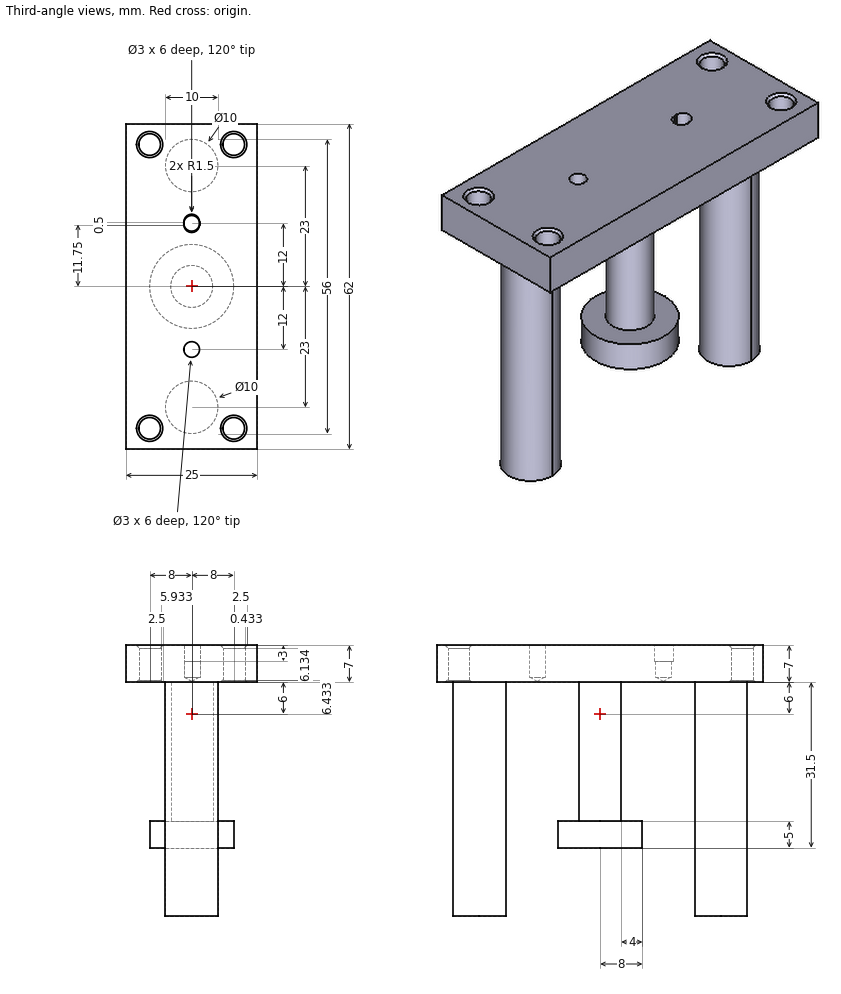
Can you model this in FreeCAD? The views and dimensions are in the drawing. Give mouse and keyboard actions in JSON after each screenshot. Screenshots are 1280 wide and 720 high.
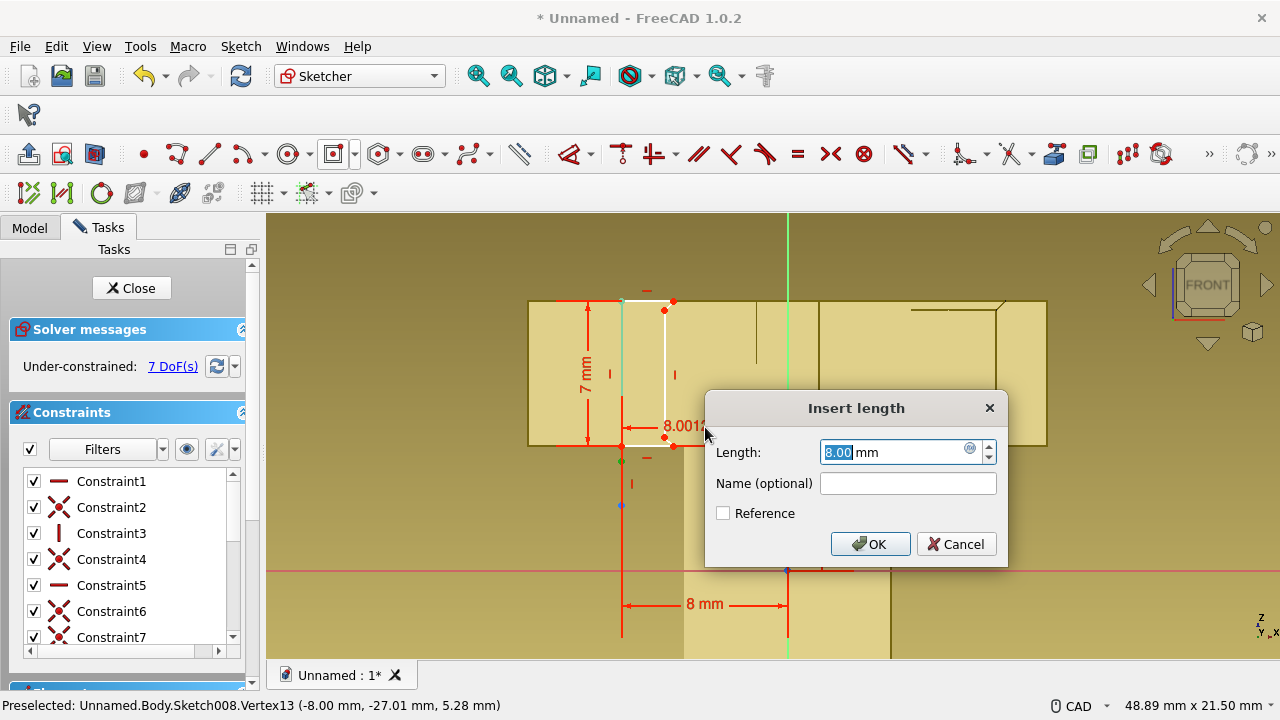
{"action": "type", "text": "8"}
{"action": "key", "text": "Return"}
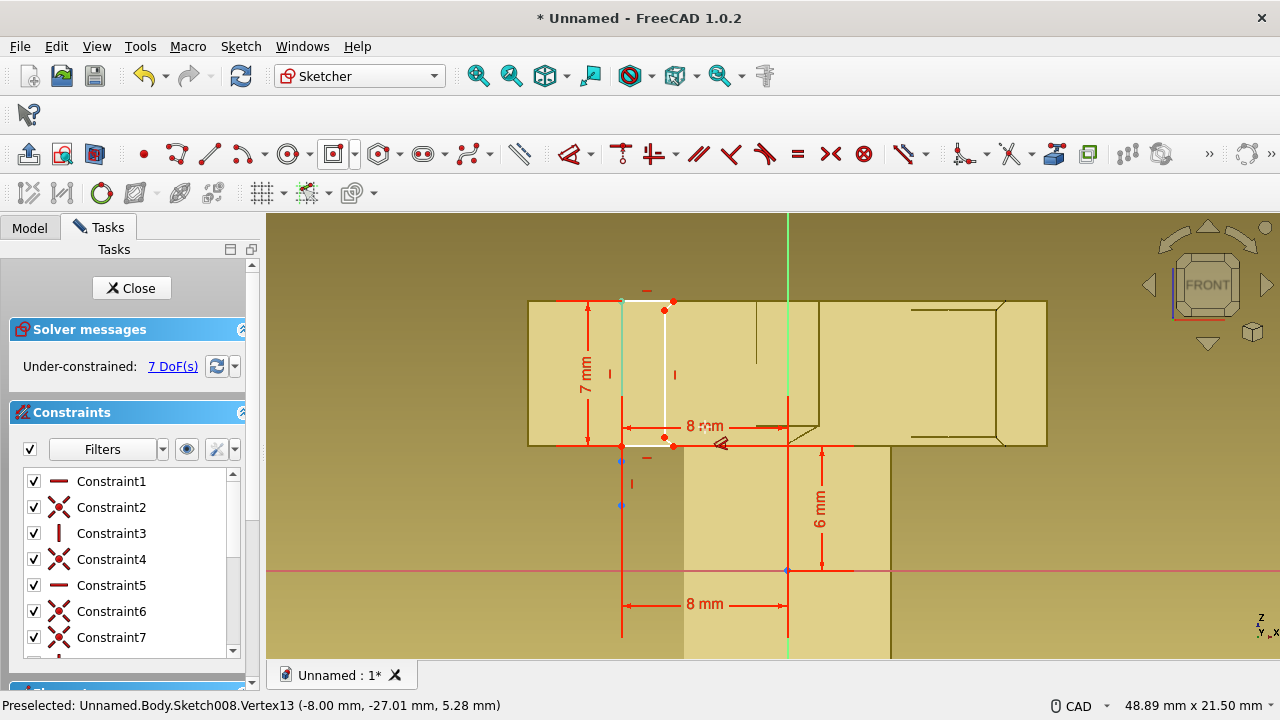
{"action": "scroll", "coordinate": [658, 446], "scroll_direction": "up", "scroll_amount": 2}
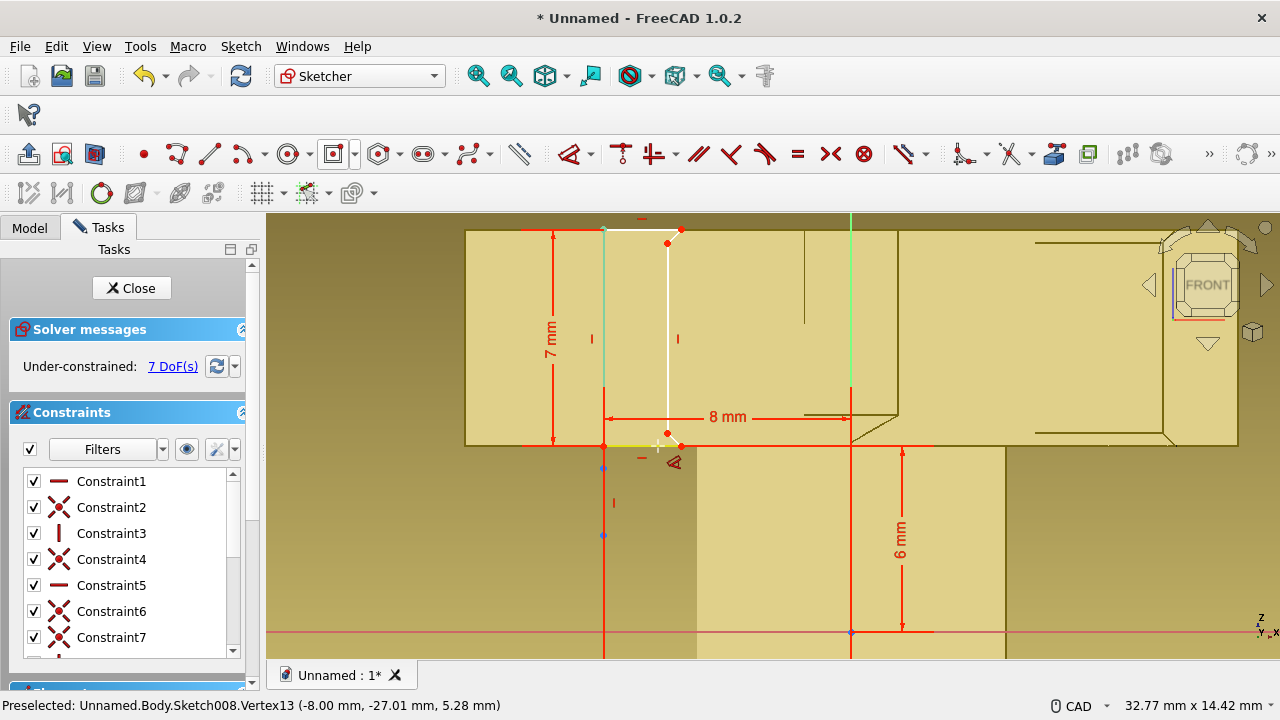
{"action": "left_click", "coordinate": [658, 446]}
{"action": "left_click", "coordinate": [643, 480]}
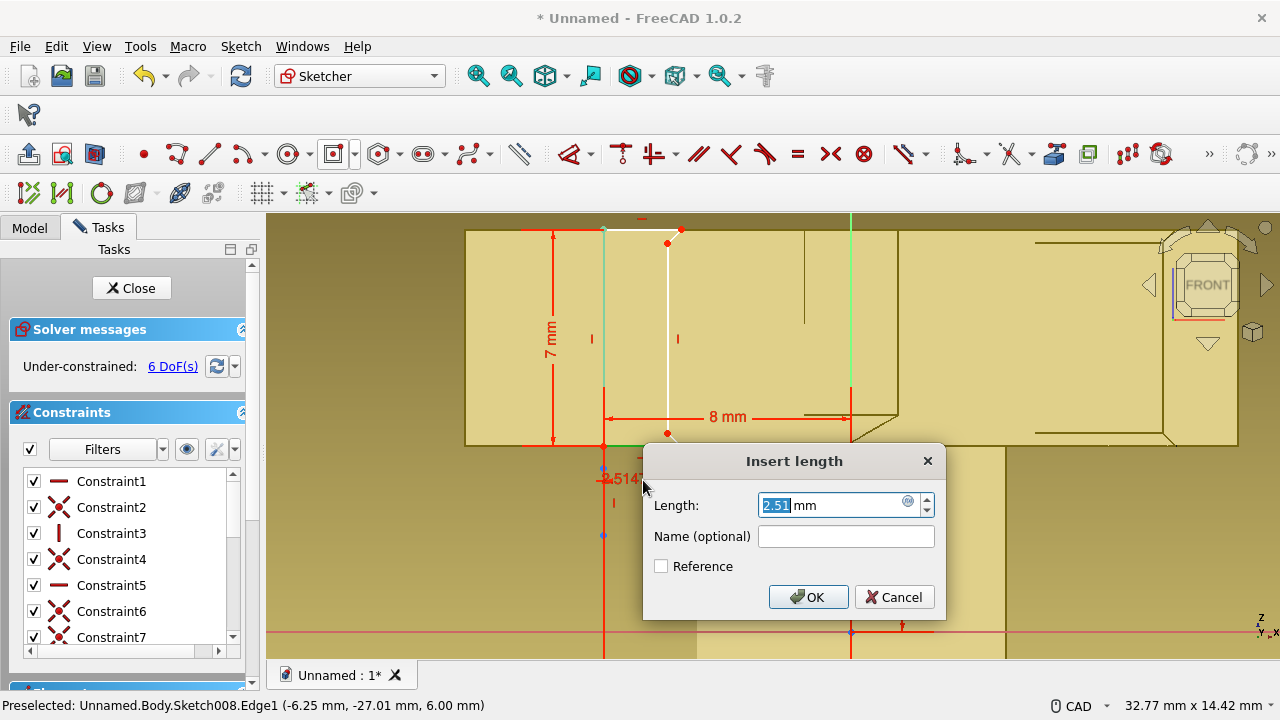
{"action": "type", "text": "2.5"}
{"action": "key", "text": "Return"}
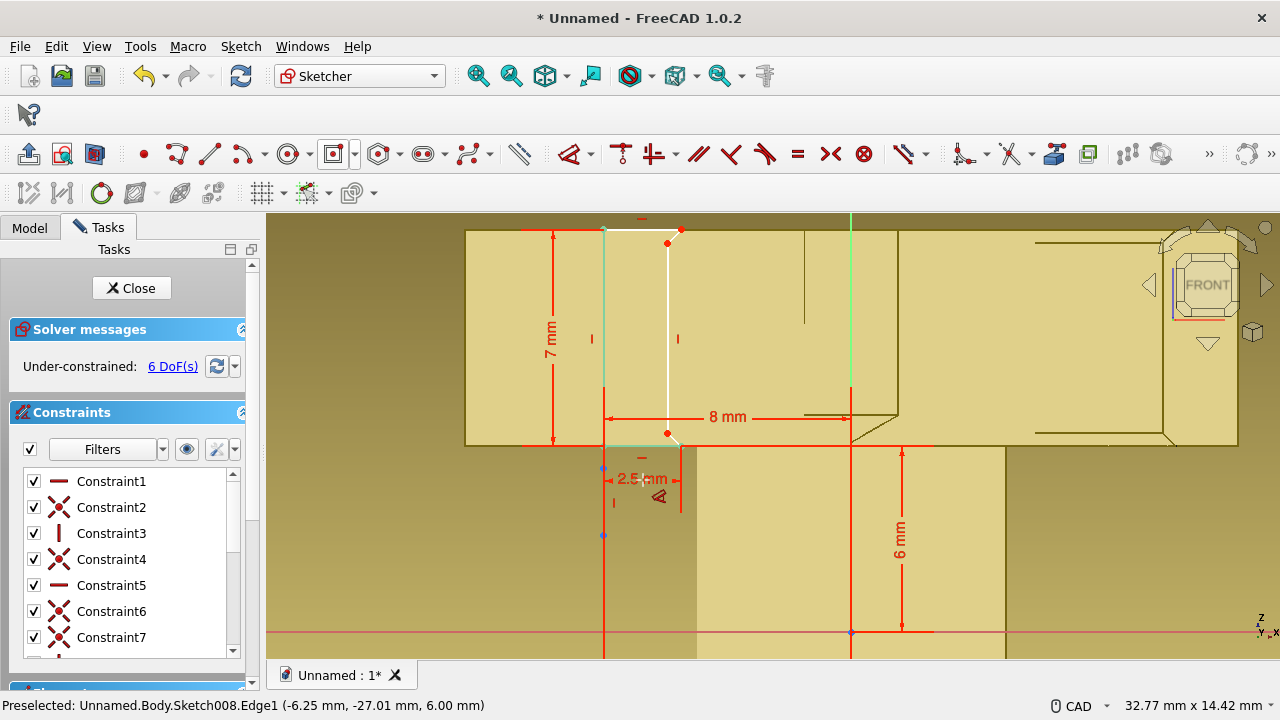
{"action": "scroll", "coordinate": [658, 446], "scroll_direction": "down", "scroll_amount": 2}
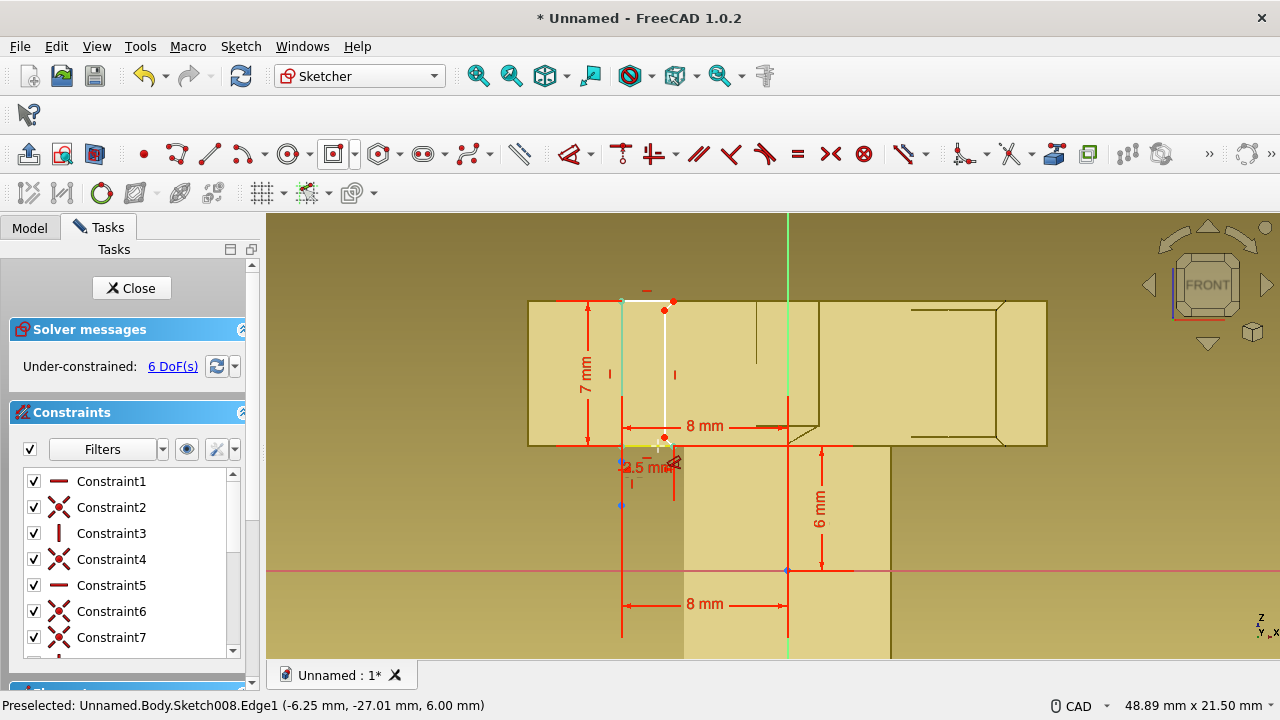
{"action": "left_click", "coordinate": [637, 301]}
{"action": "left_click", "coordinate": [648, 267]}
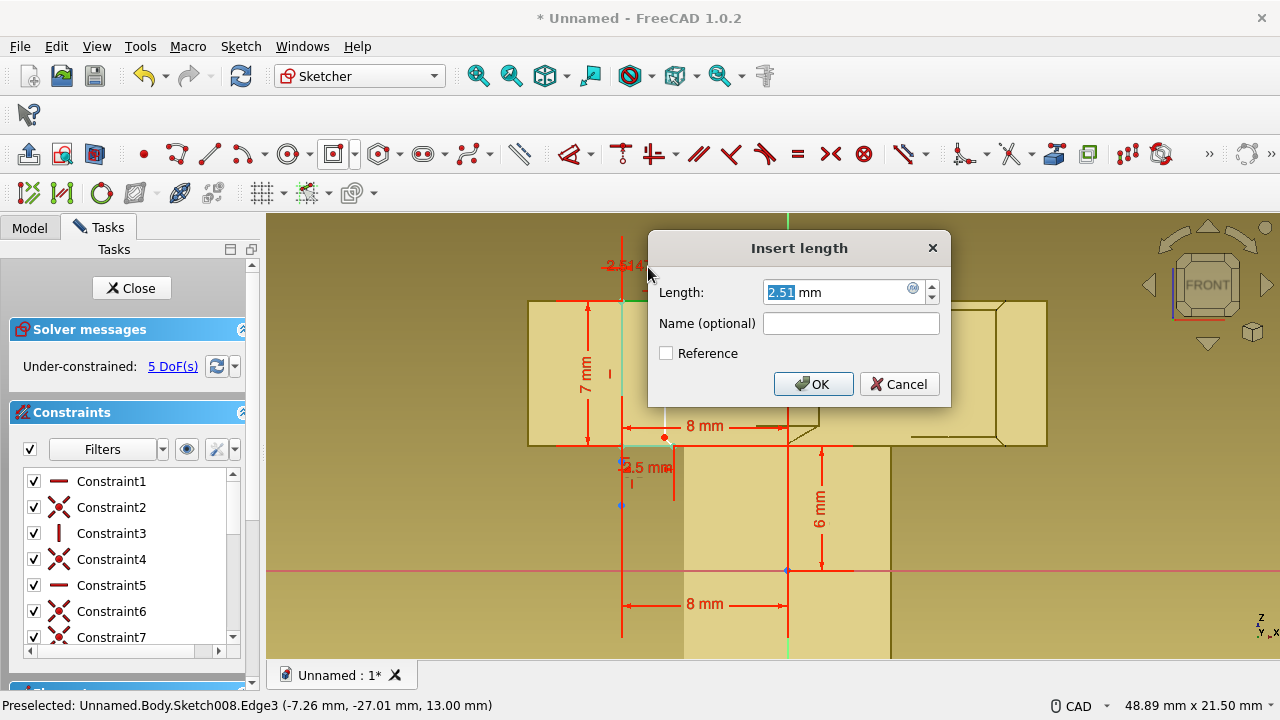
{"action": "type", "text": "2.5"}
{"action": "key", "text": "Return"}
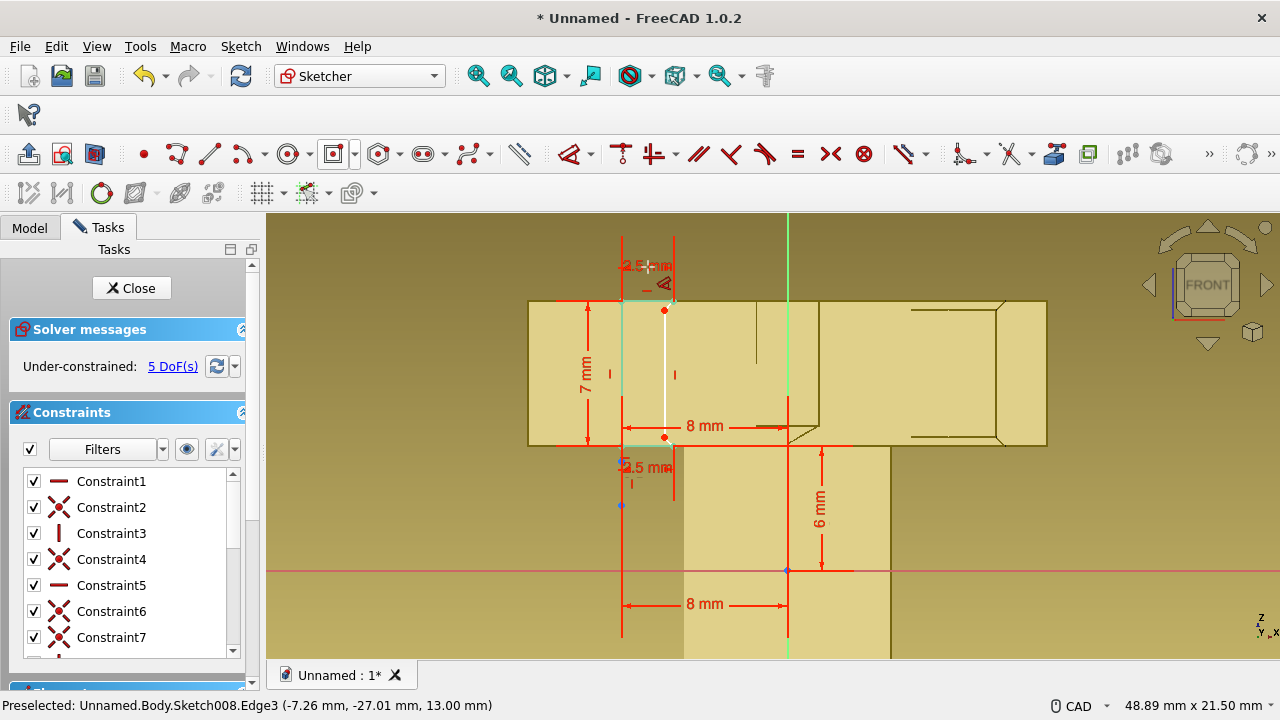
{"action": "left_click", "coordinate": [665, 349]}
{"action": "left_click", "coordinate": [699, 374]}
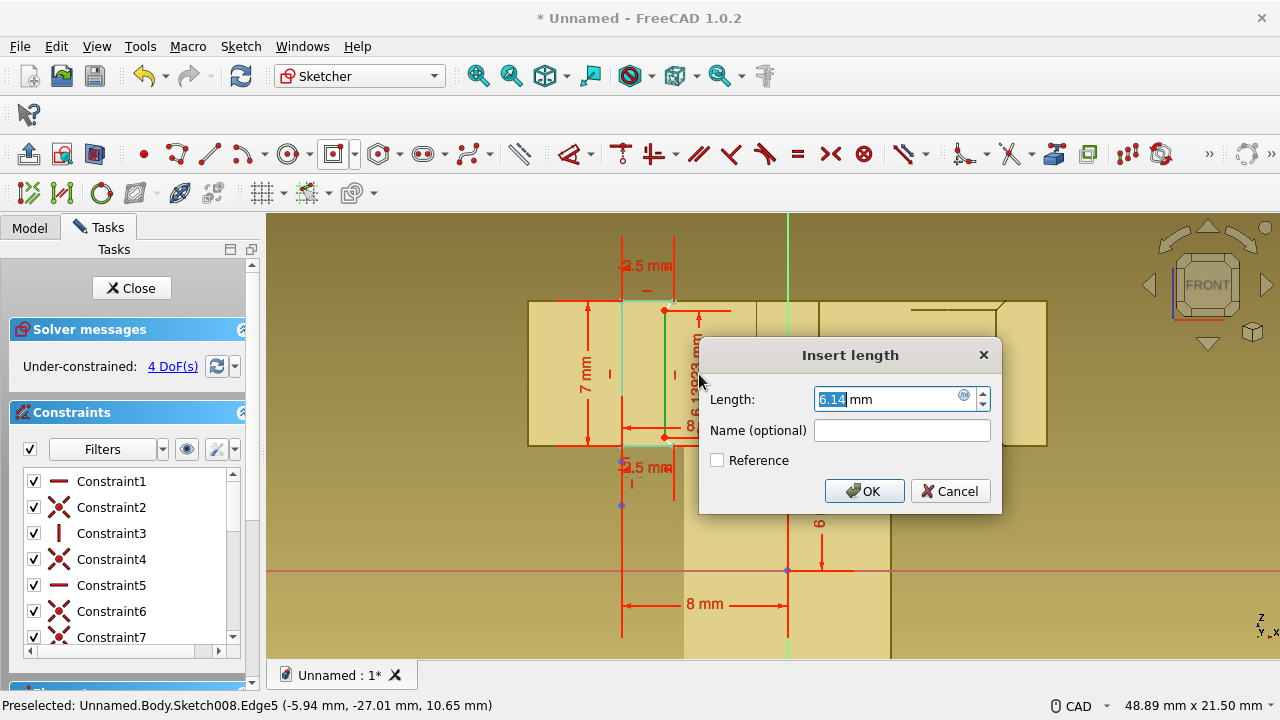
{"action": "type", "text": "6.134"}
{"action": "key", "text": "Return"}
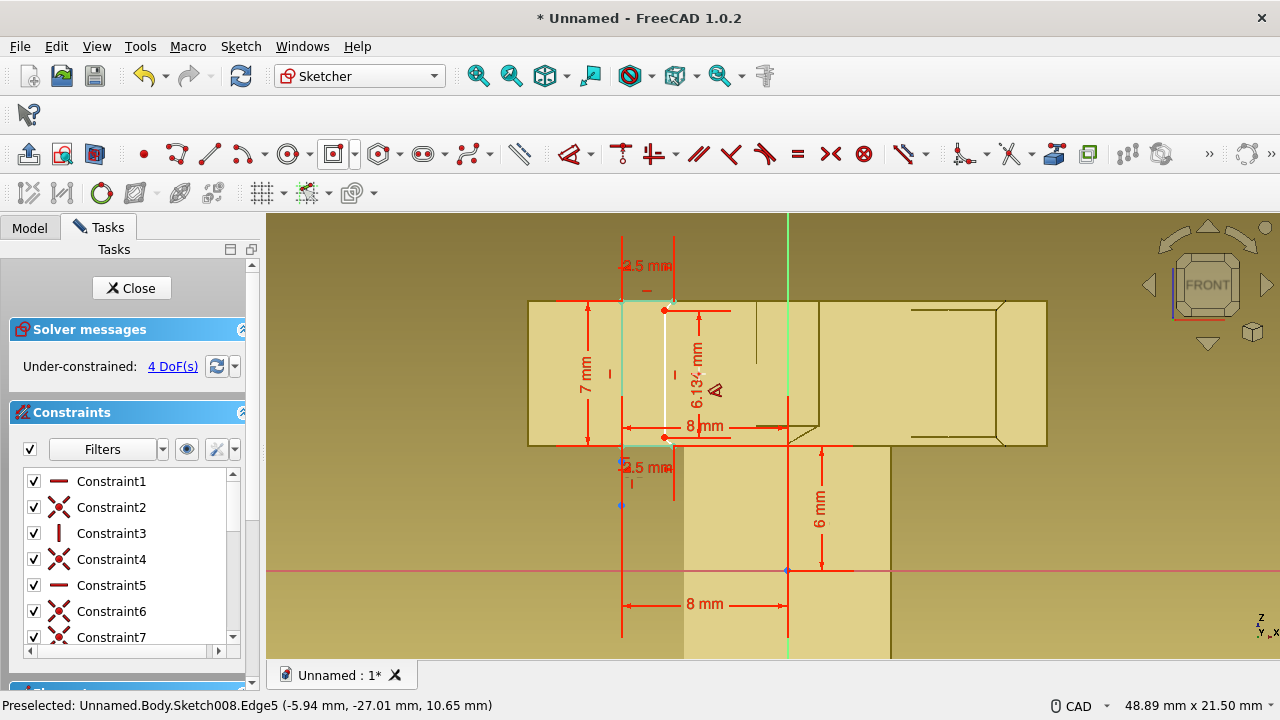
{"action": "left_click", "coordinate": [665, 311]}
{"action": "left_click", "coordinate": [726, 277]}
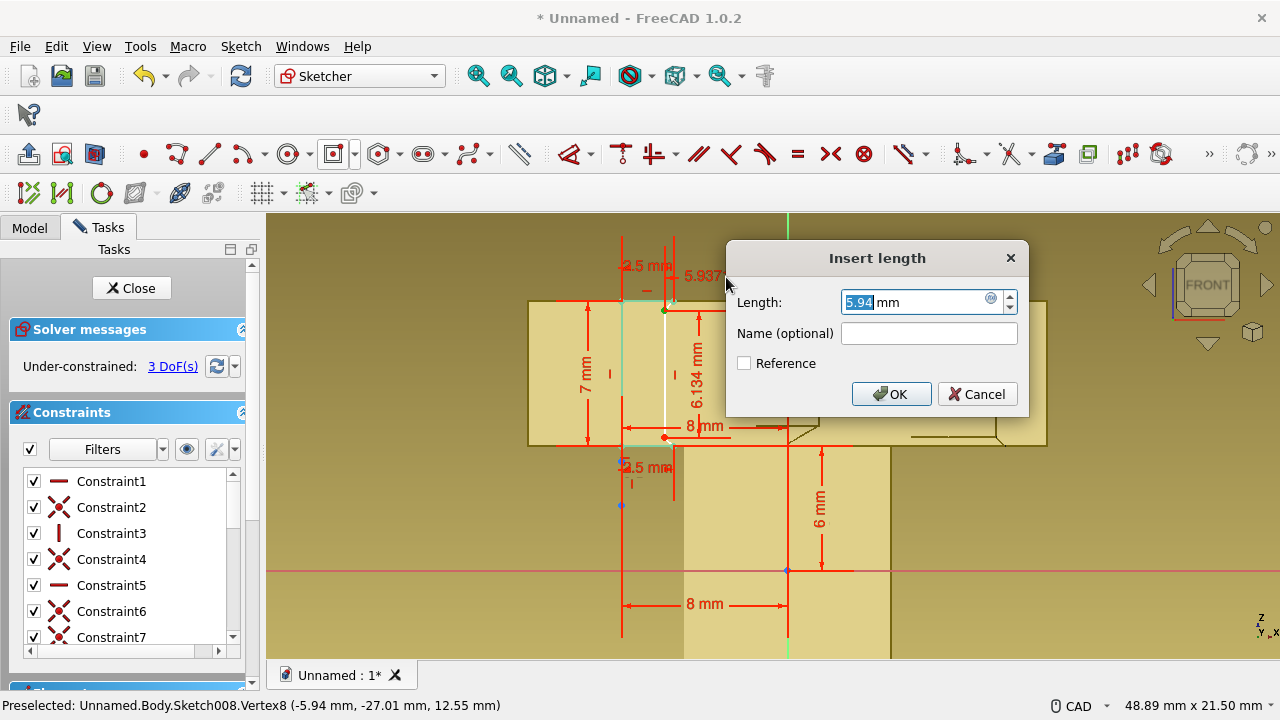
{"action": "type", "text": "5.933"}
{"action": "key", "text": "Return"}